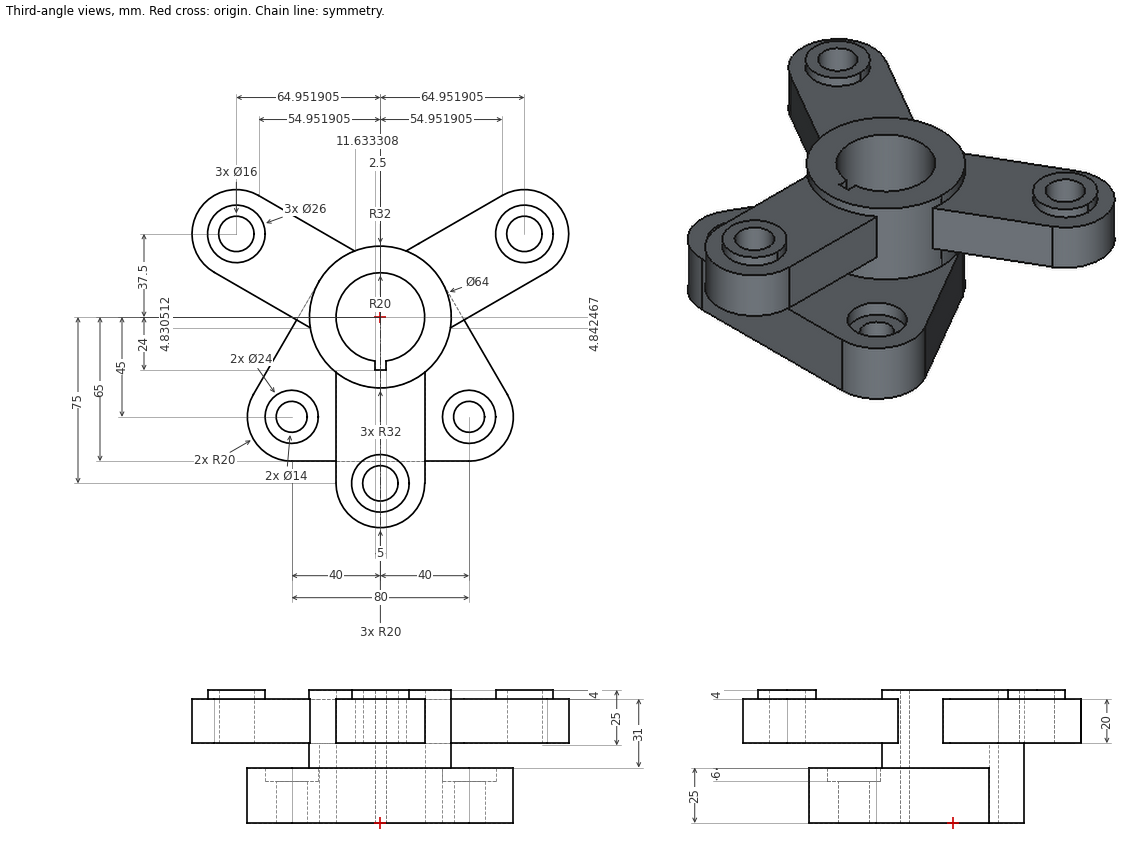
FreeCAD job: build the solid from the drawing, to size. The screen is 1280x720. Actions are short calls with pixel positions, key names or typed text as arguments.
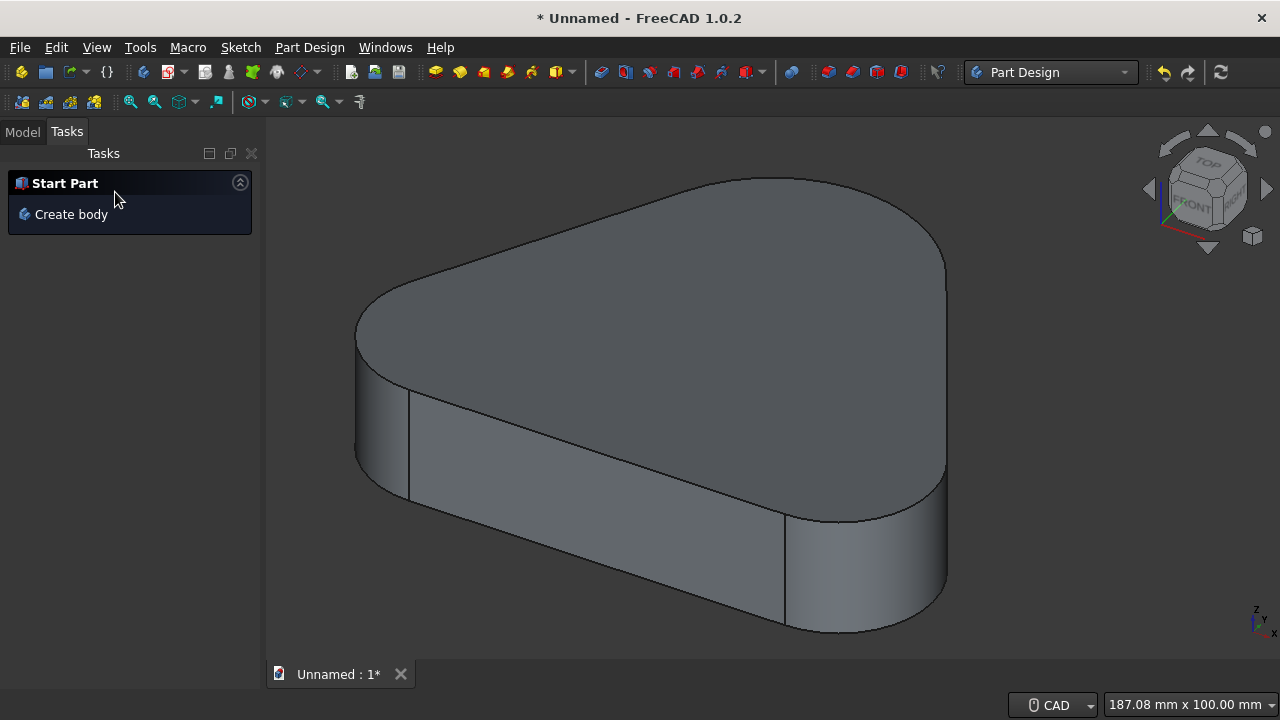
click(132, 102)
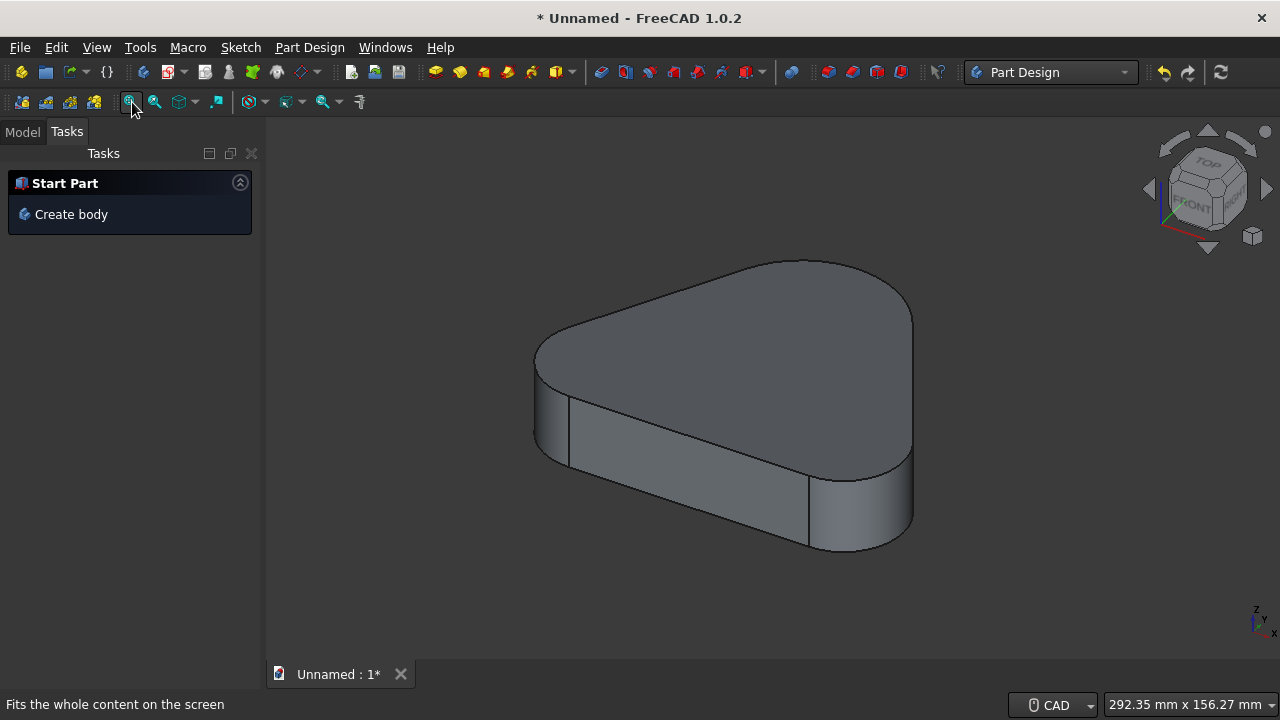
click(773, 351)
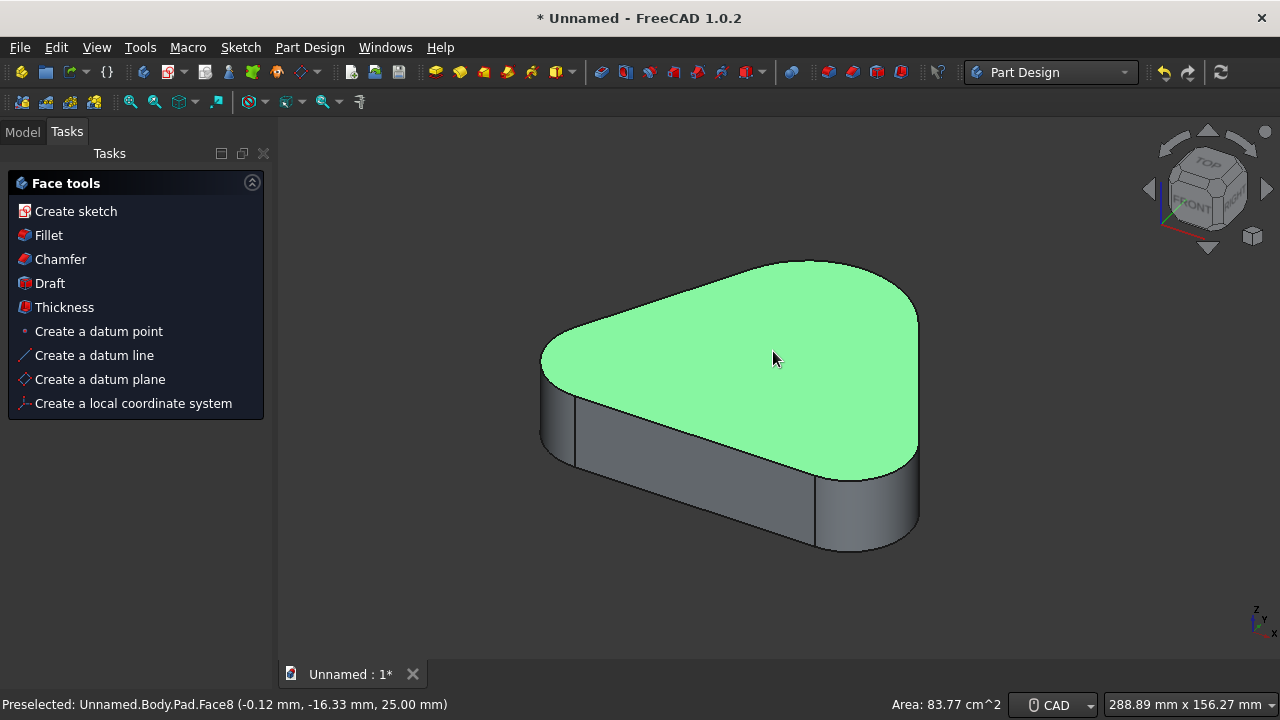
click(168, 72)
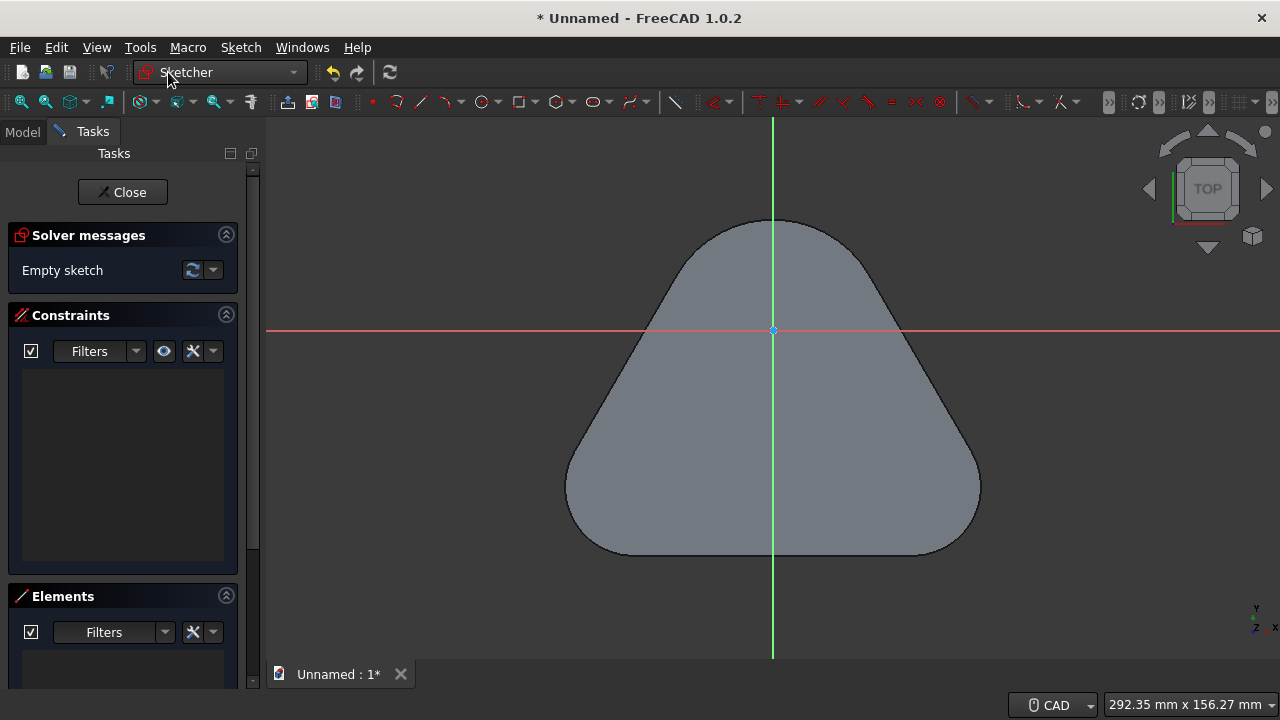
scroll(912, 214, up, 2)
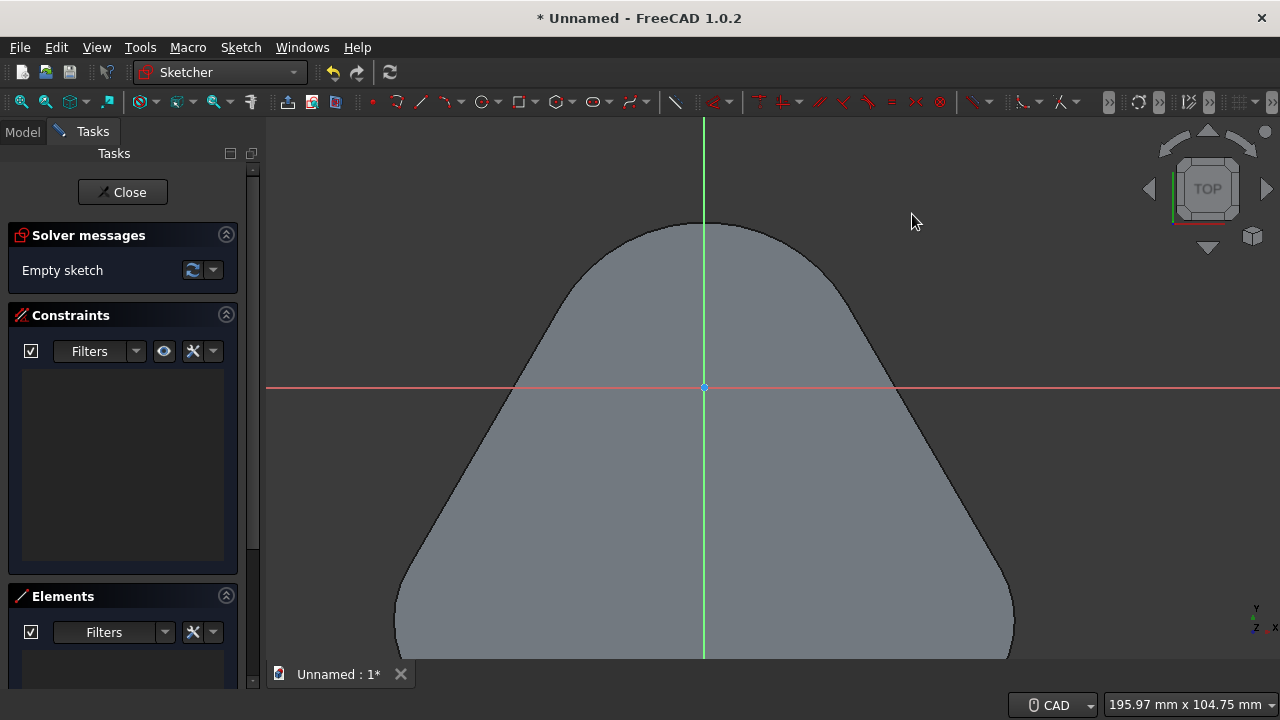
key(g)
key(c)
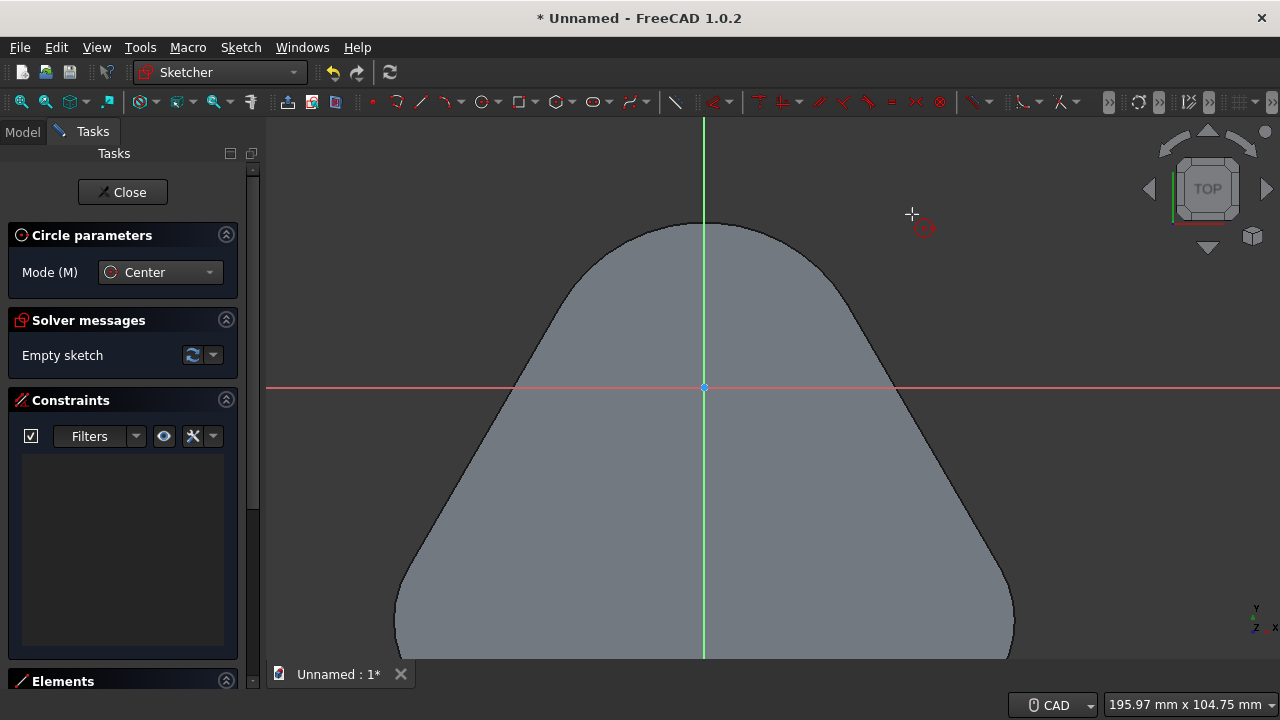
click(704, 388)
click(821, 271)
key(Escape)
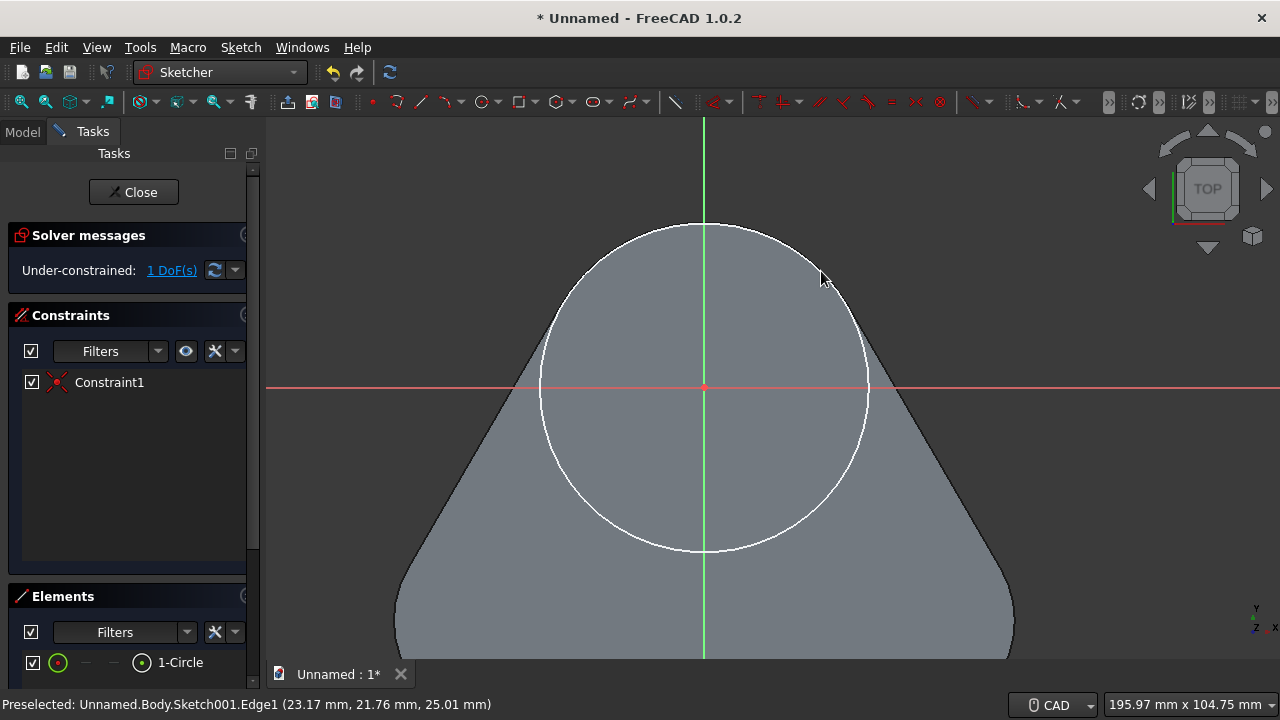
click(820, 271)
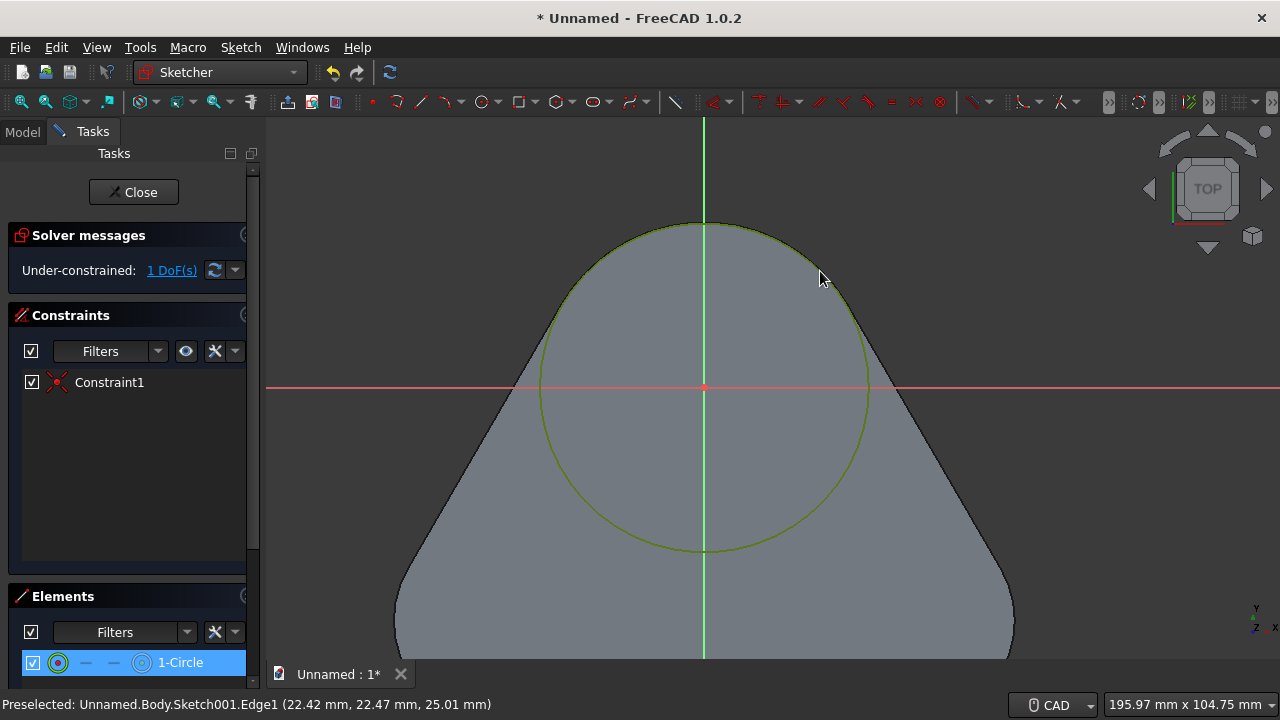
click(732, 102)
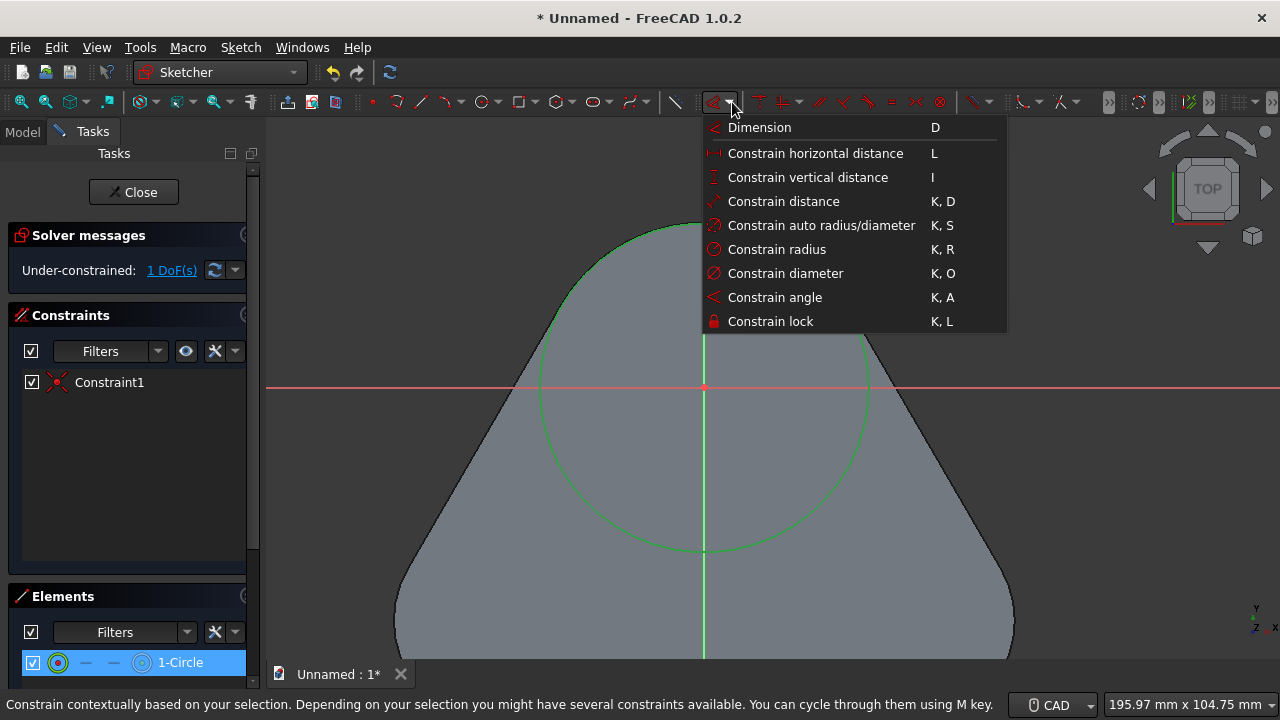
click(855, 273)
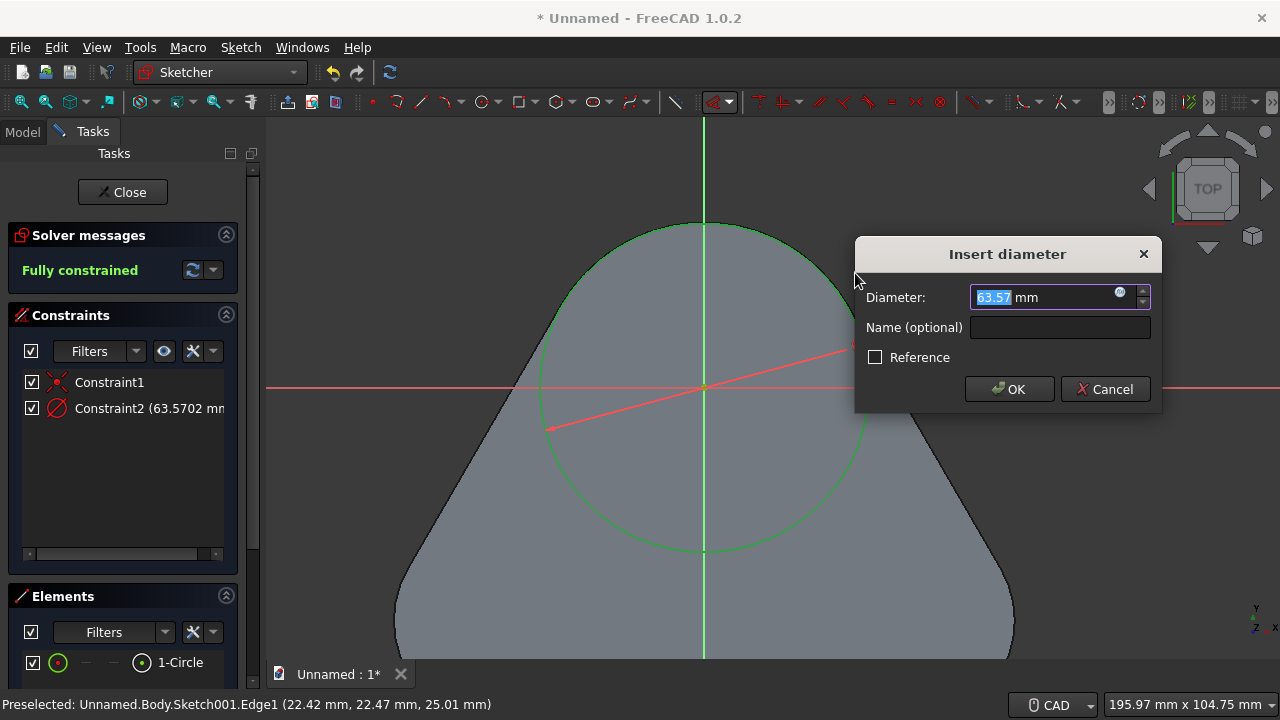
text(64)
key(Return)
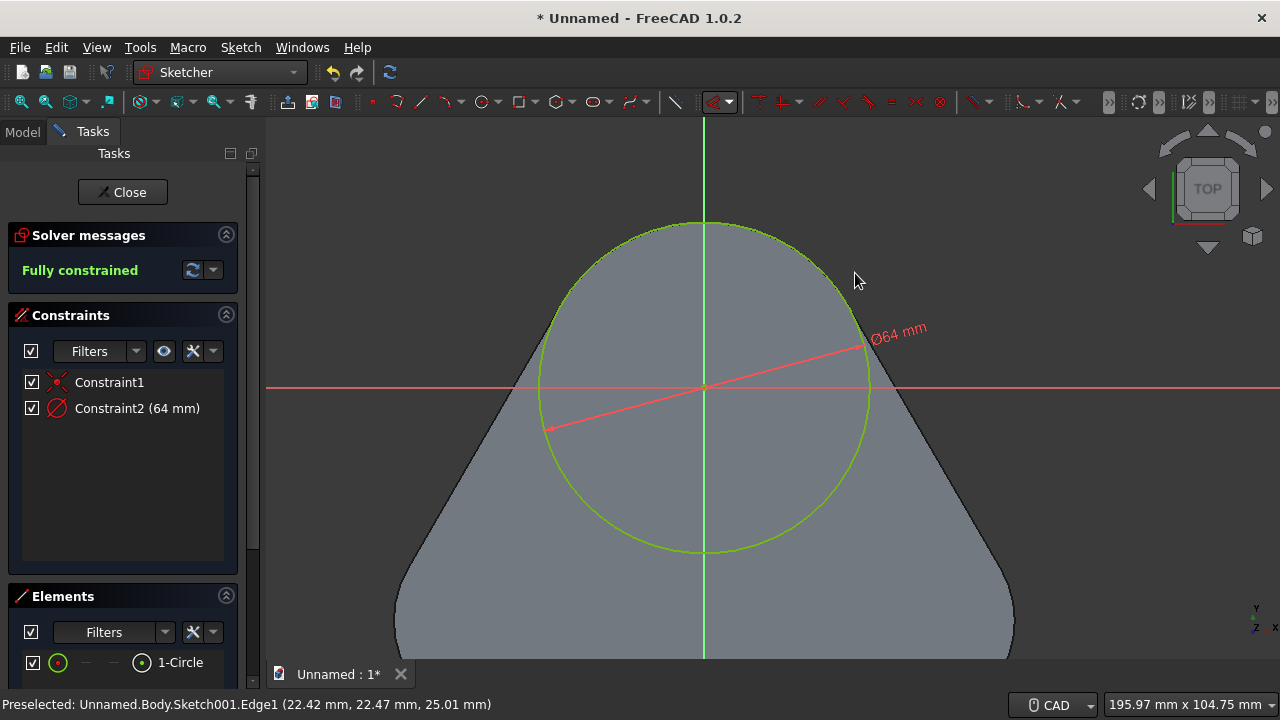
click(123, 192)